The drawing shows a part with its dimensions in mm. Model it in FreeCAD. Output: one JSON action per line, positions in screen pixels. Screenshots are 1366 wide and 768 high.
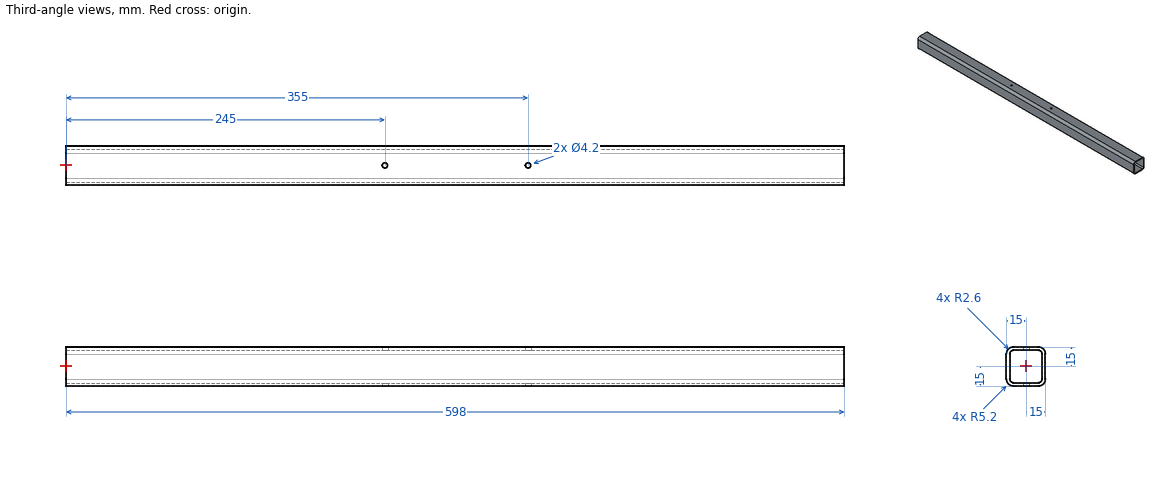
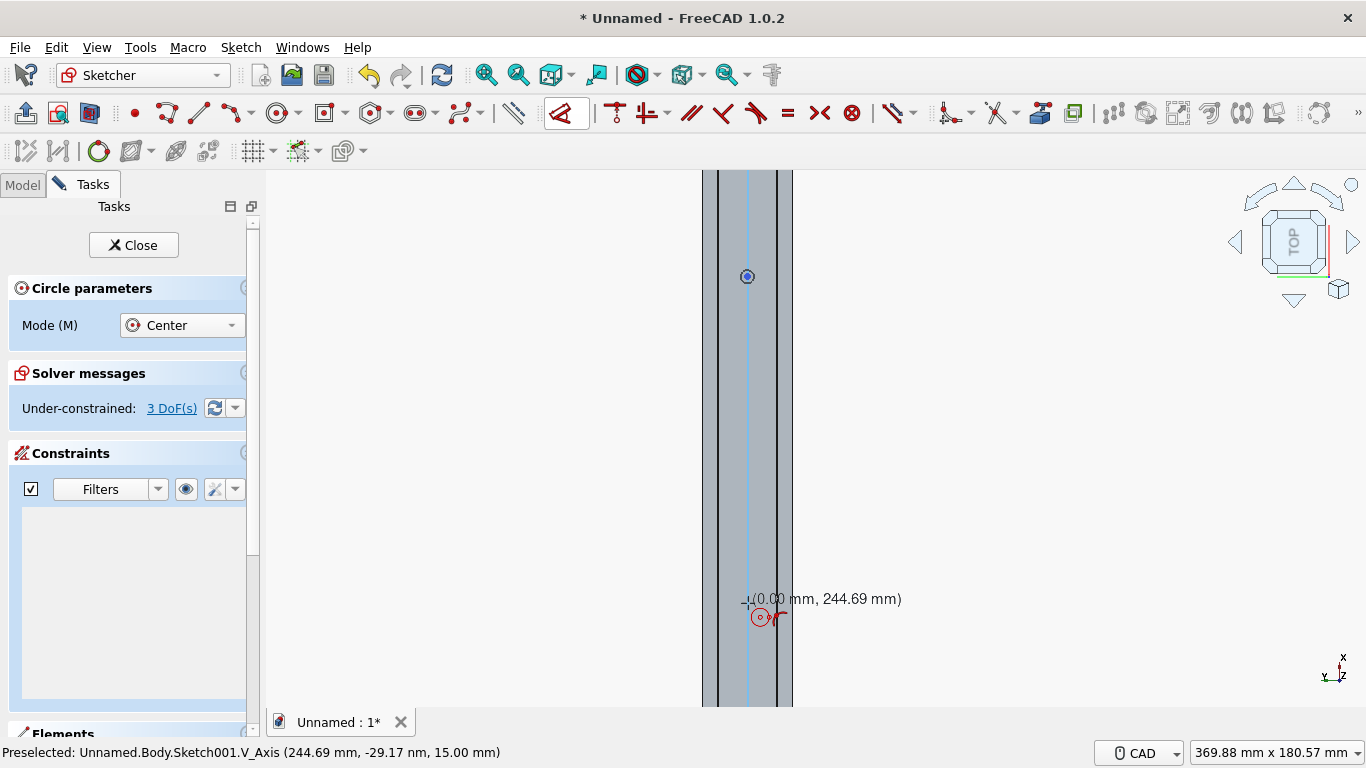
{"action": "left_click", "coordinate": [748, 603]}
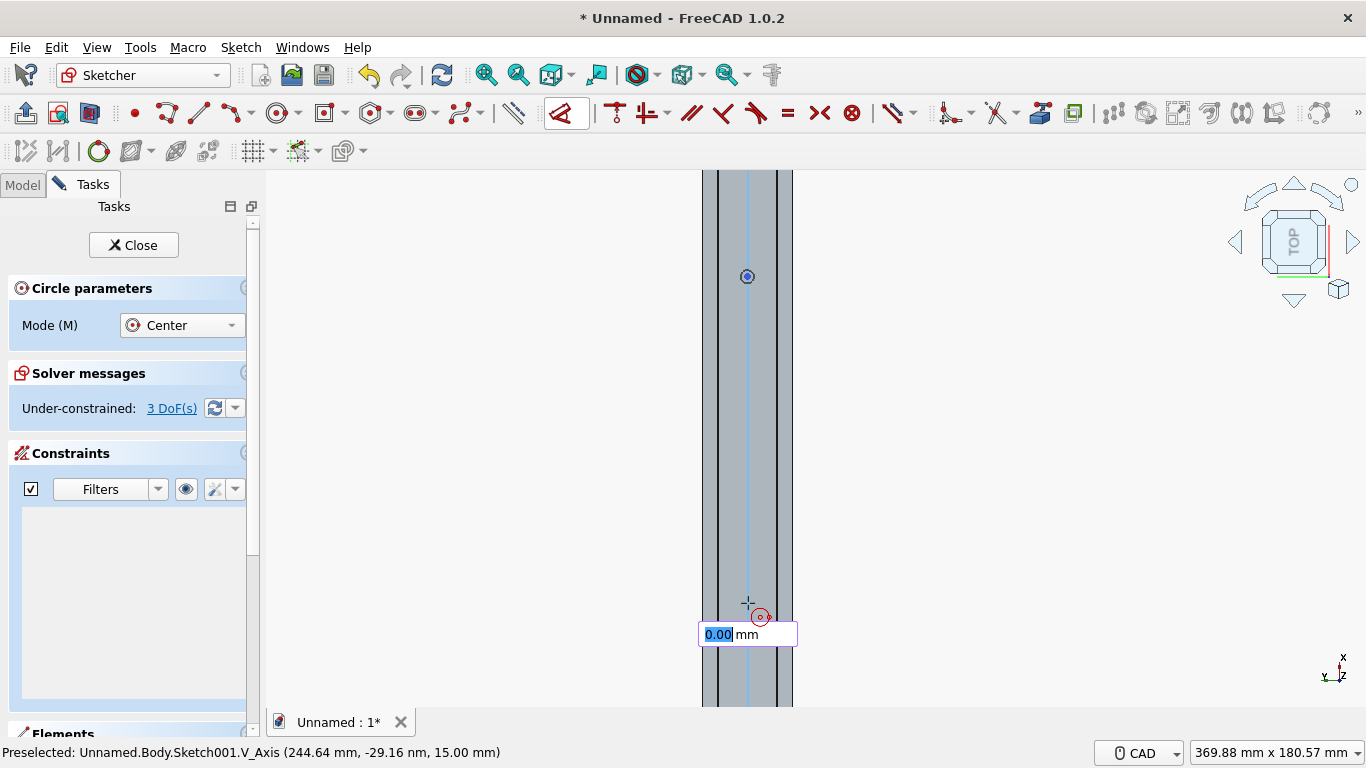
{"action": "scroll", "coordinate": [753, 601], "scroll_direction": "up", "scroll_amount": 5}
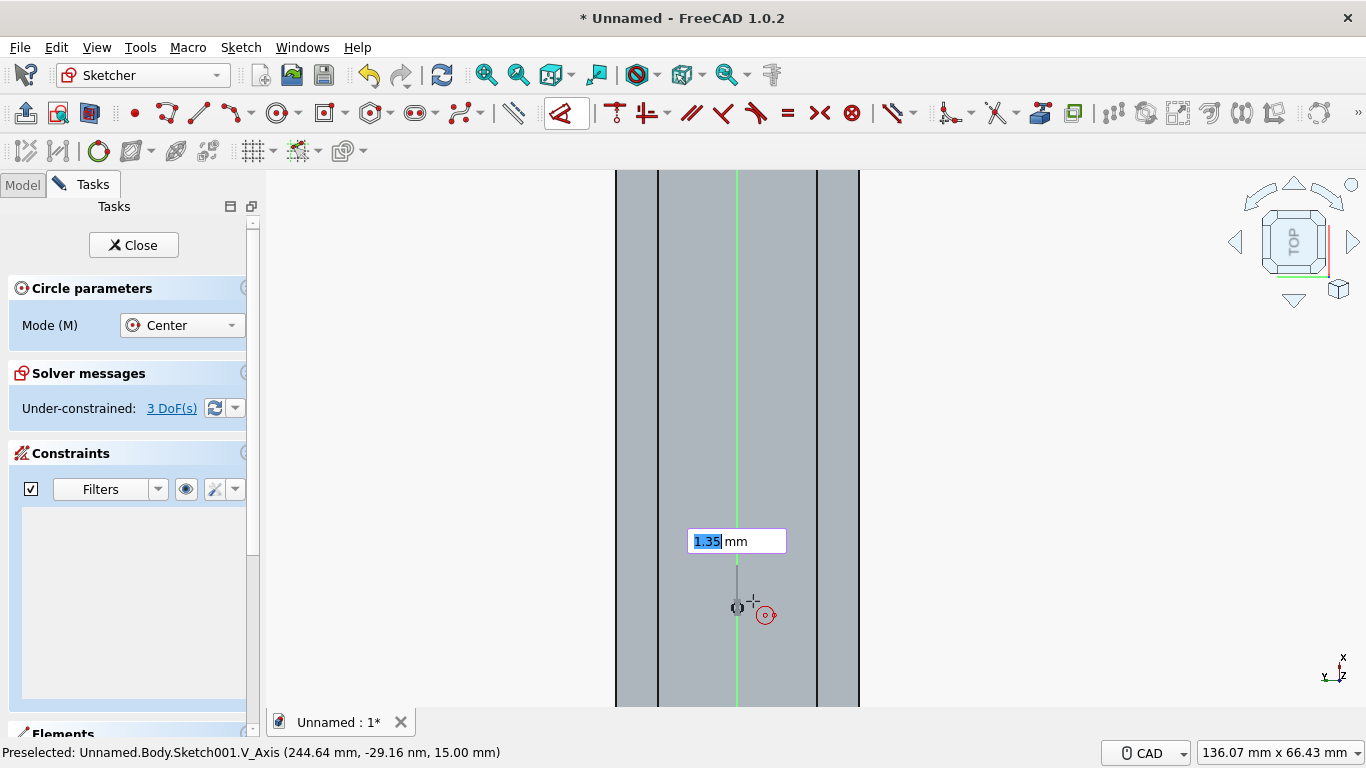
{"action": "left_click", "coordinate": [753, 599]}
{"action": "key", "text": "Escape"}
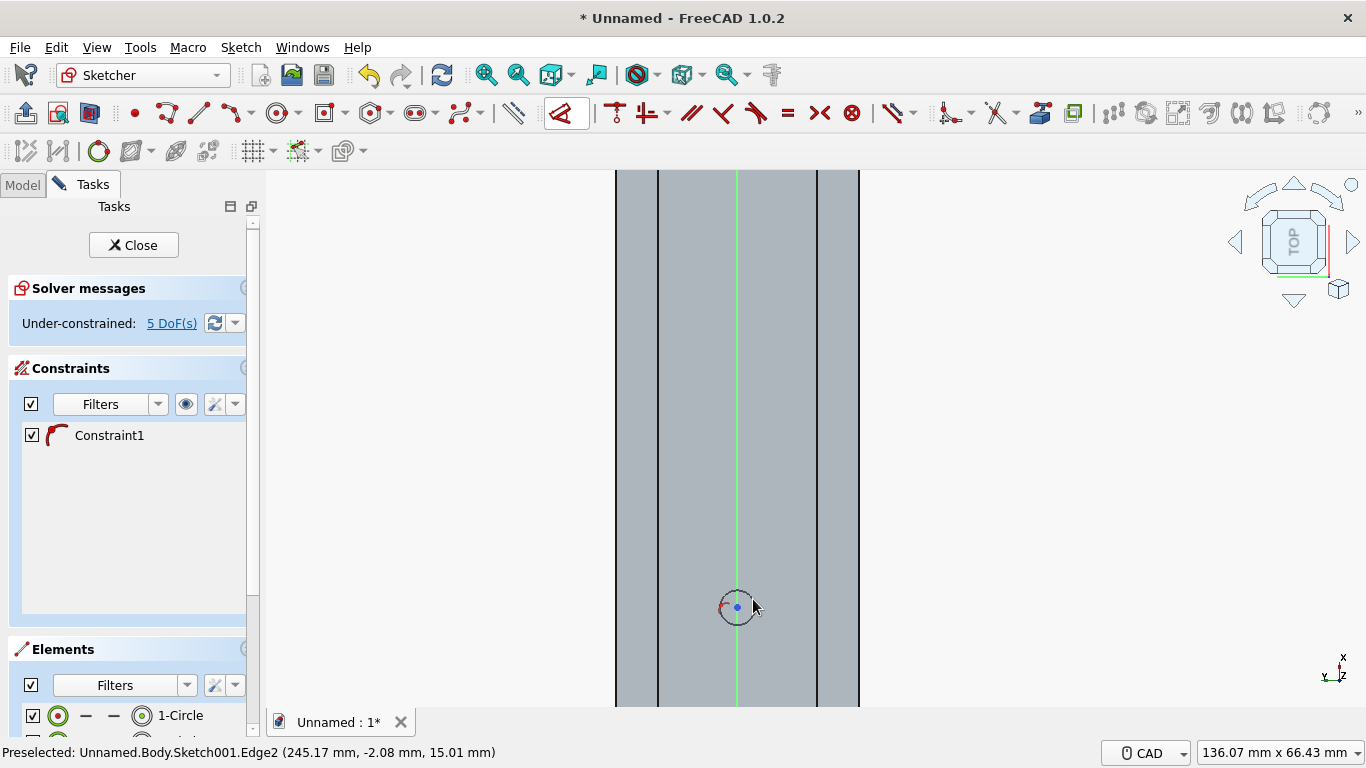
{"action": "scroll", "coordinate": [753, 600], "scroll_direction": "down", "scroll_amount": 5}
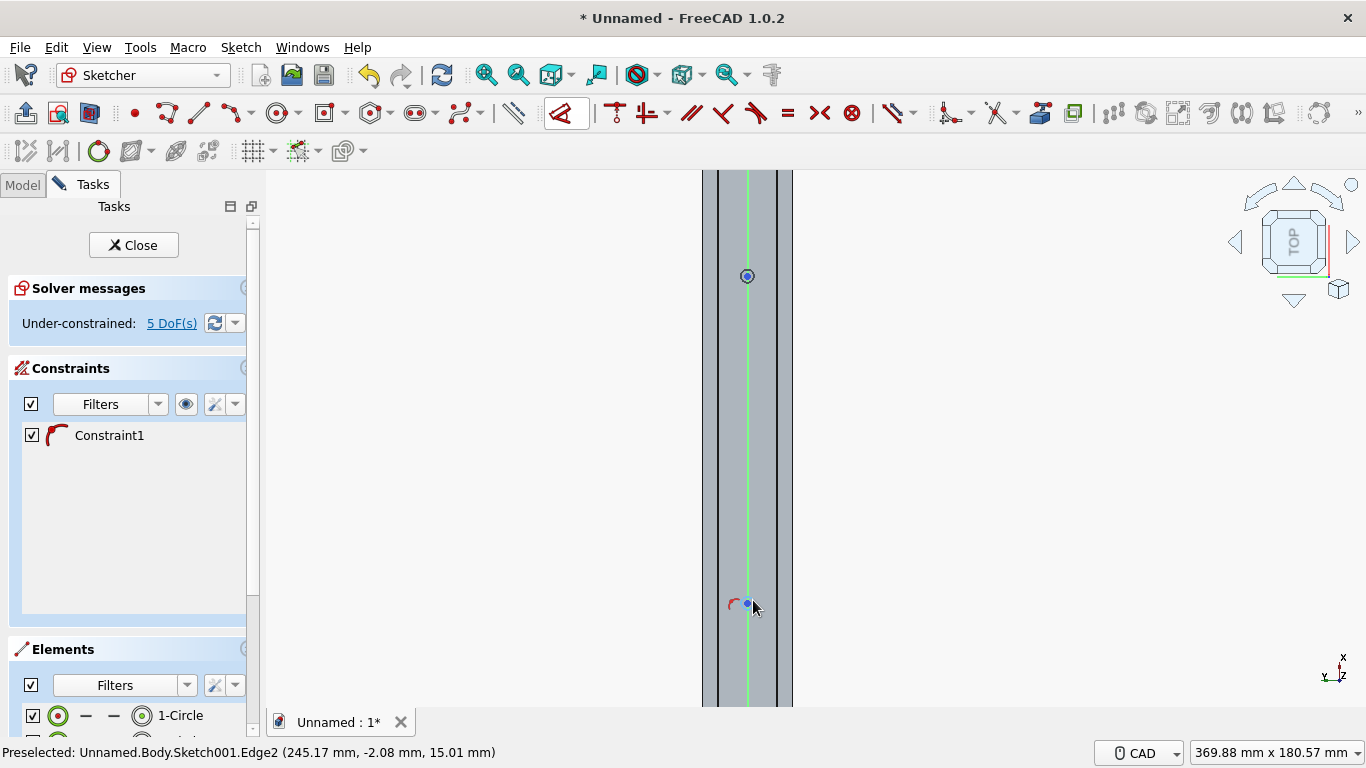
{"action": "scroll", "coordinate": [752, 271], "scroll_direction": "up", "scroll_amount": 6}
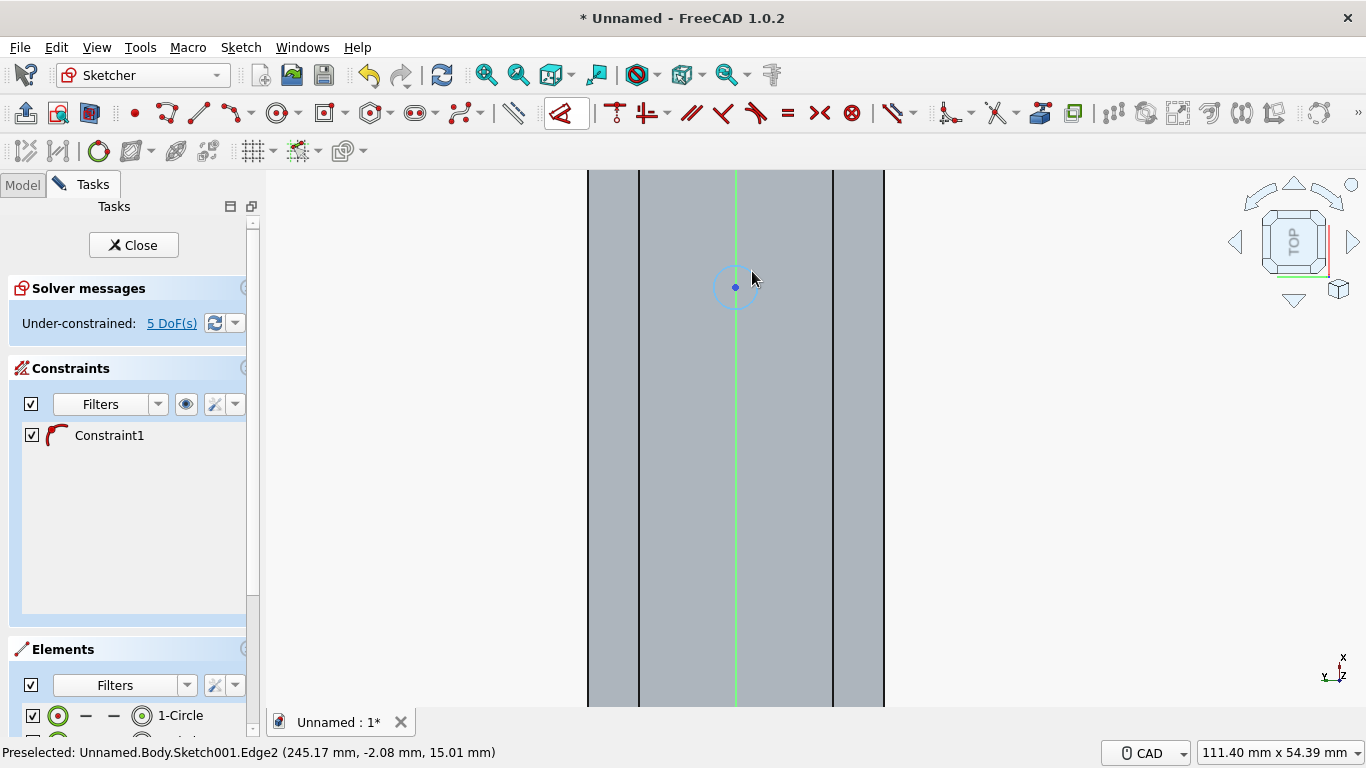
{"action": "left_click", "coordinate": [751, 272]}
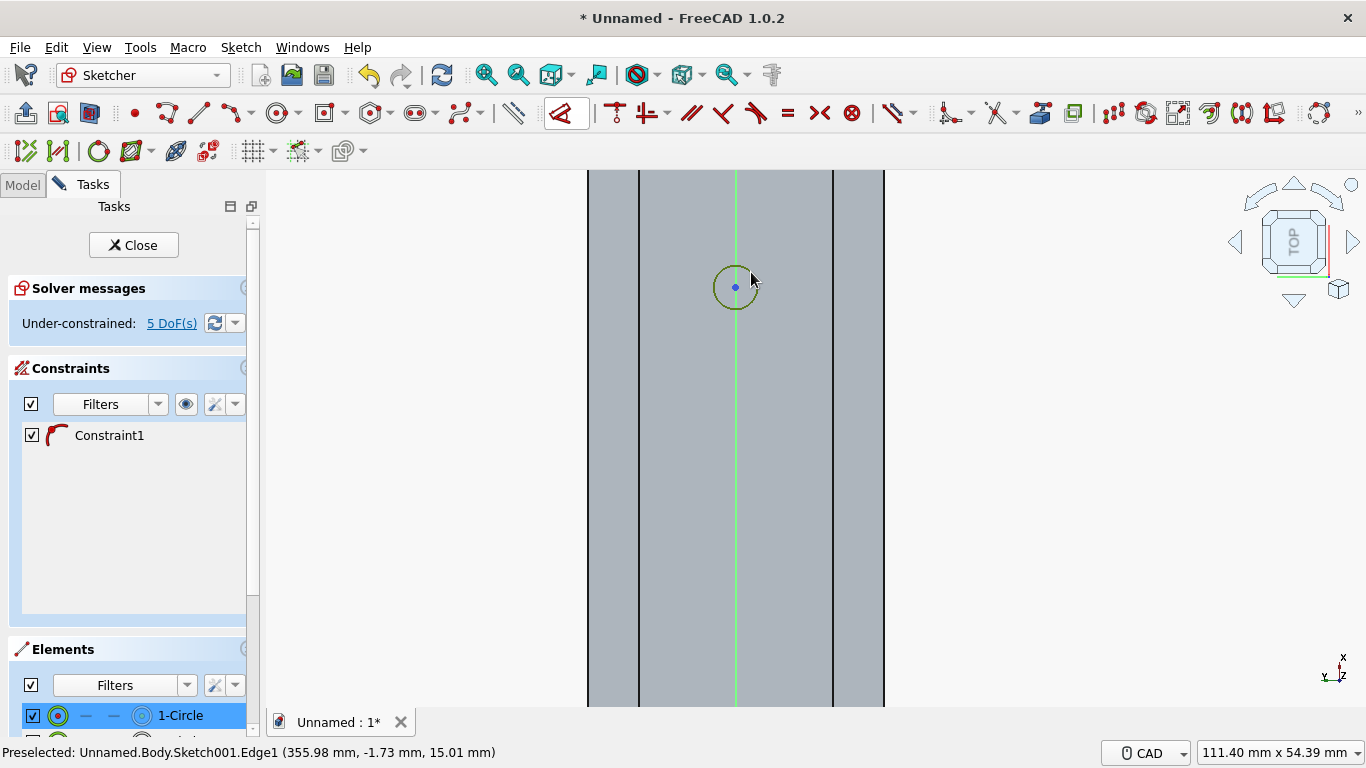
{"action": "scroll", "coordinate": [752, 271], "scroll_direction": "down", "scroll_amount": 6}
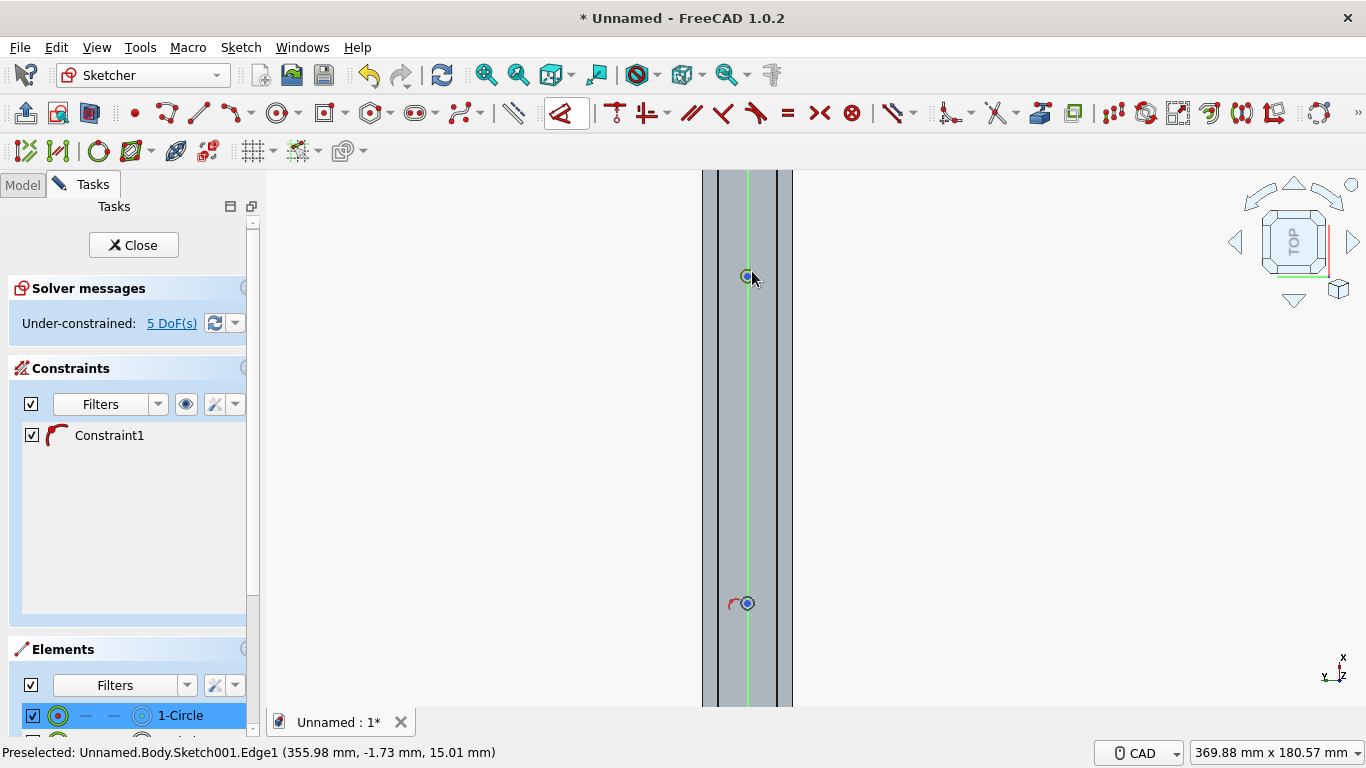
{"action": "scroll", "coordinate": [752, 599], "scroll_direction": "up", "scroll_amount": 6}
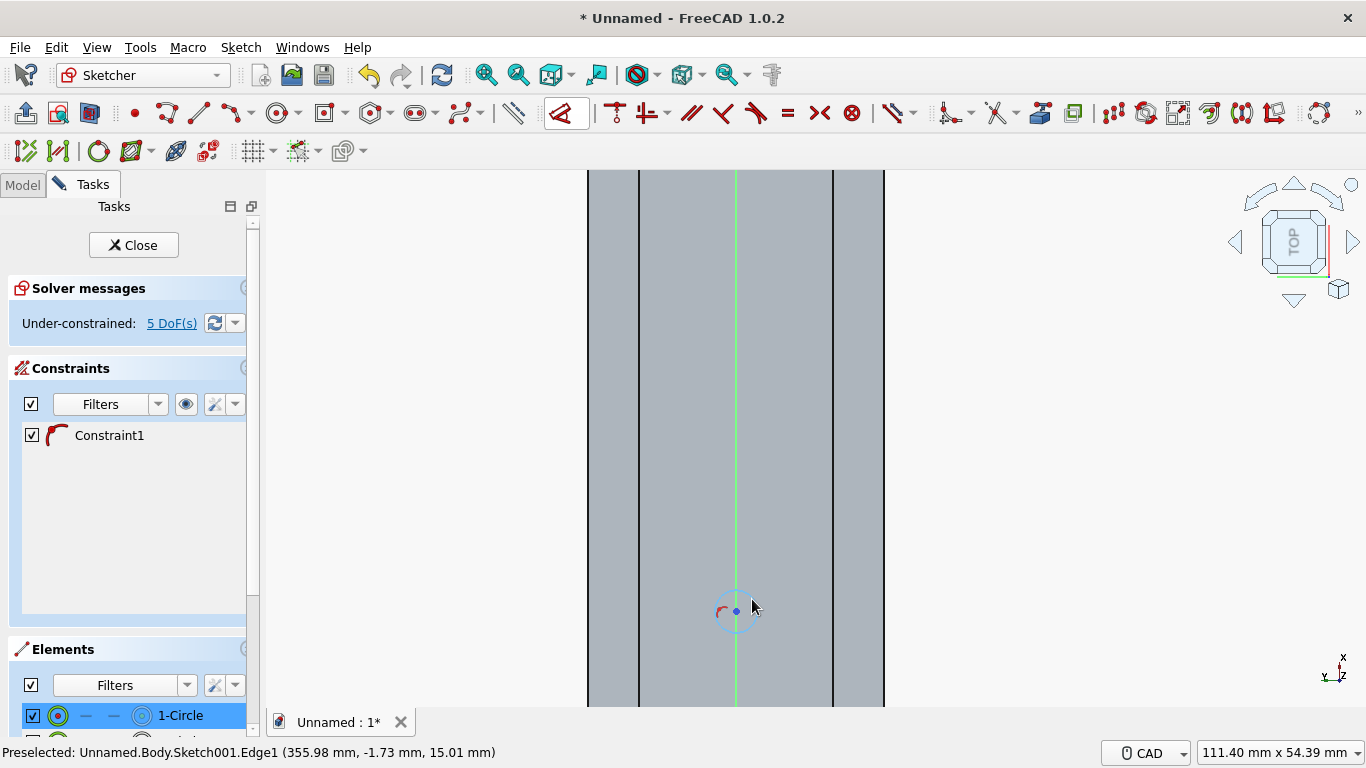
{"action": "left_click", "coordinate": [751, 597]}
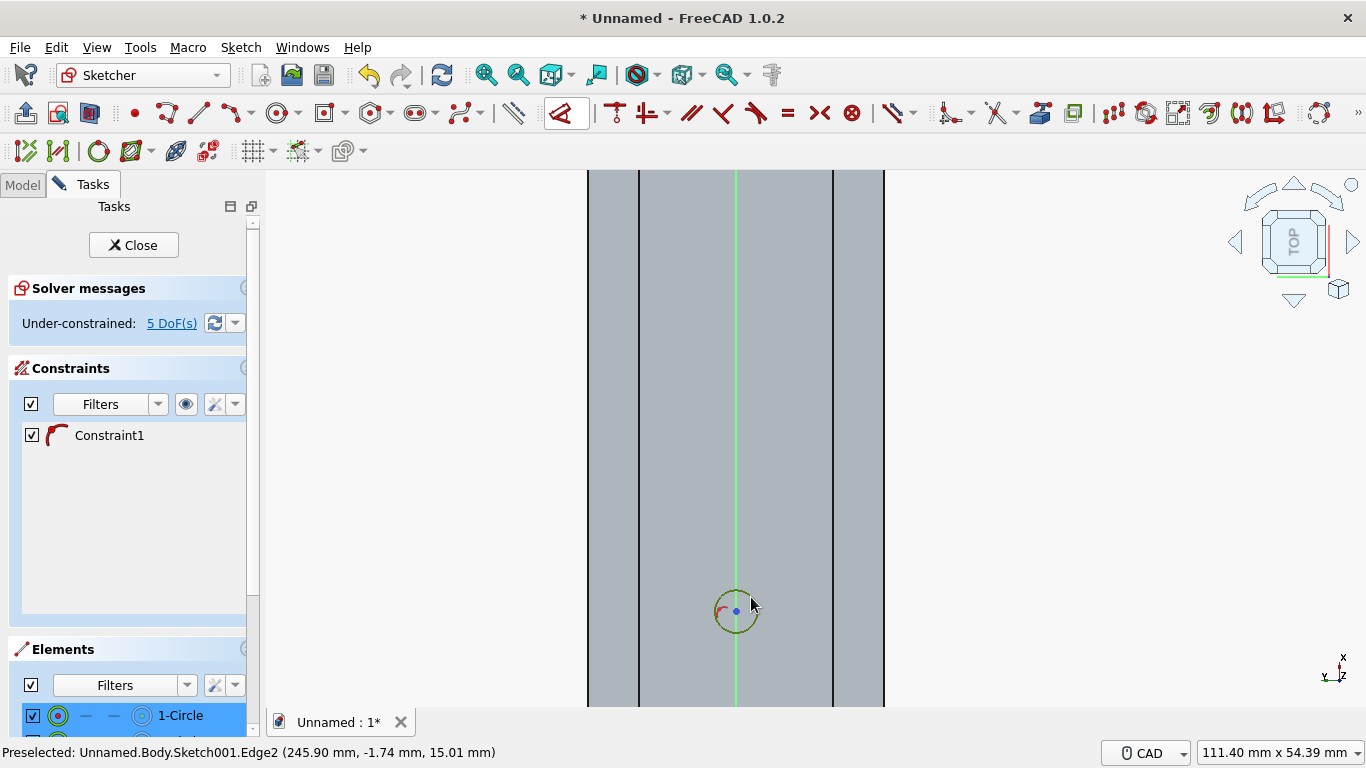
{"action": "key", "text": "e"}